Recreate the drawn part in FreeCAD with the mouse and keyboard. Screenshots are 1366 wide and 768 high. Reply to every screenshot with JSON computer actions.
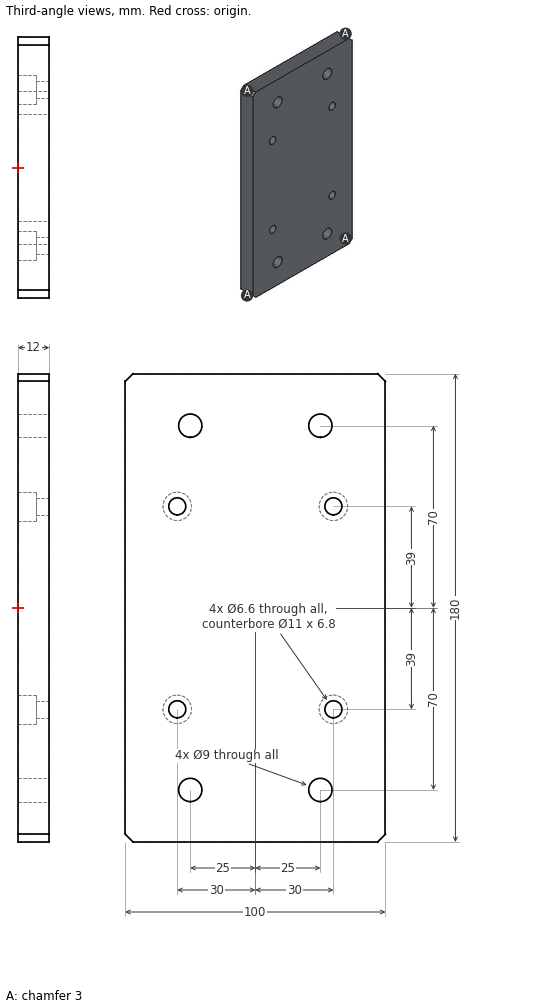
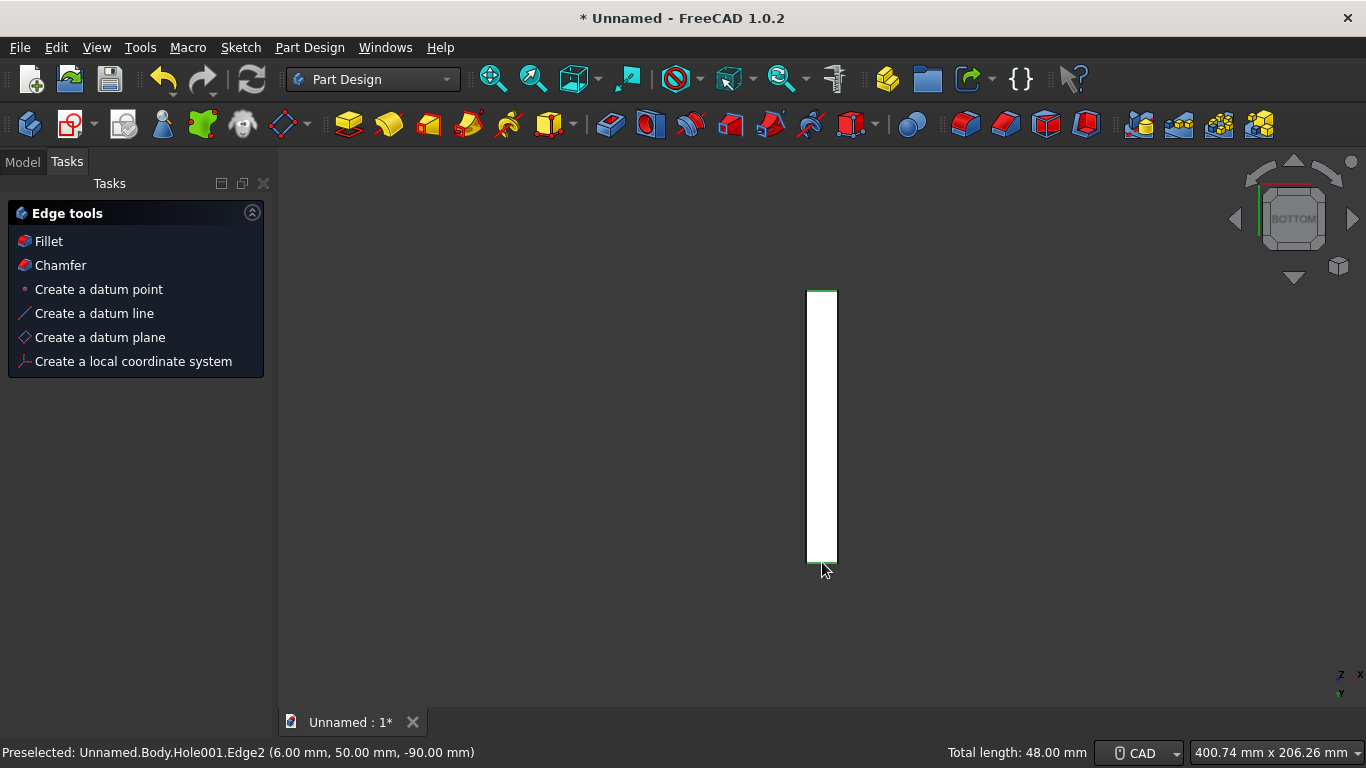
{"action": "left_click", "coordinate": [1006, 124]}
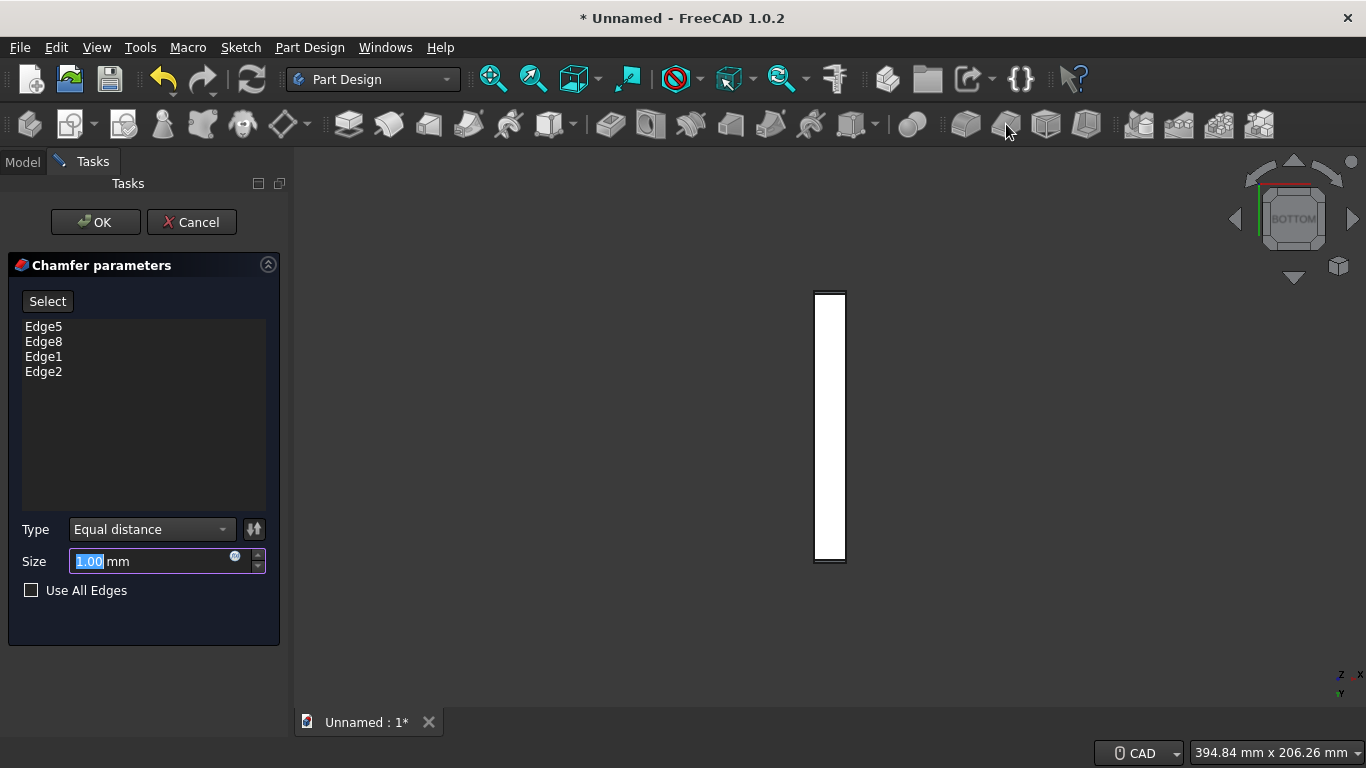
{"action": "type", "text": "3"}
{"action": "key", "text": "Tab"}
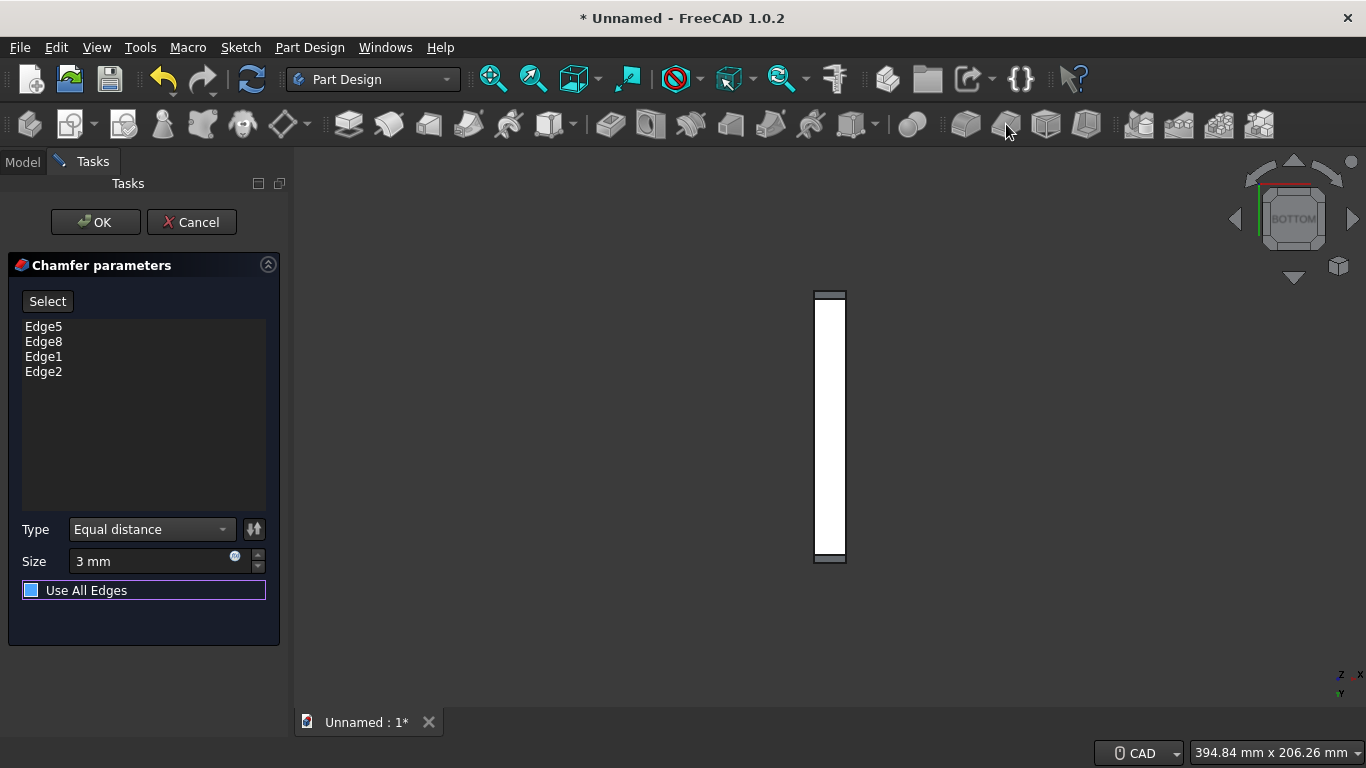
{"action": "left_click", "coordinate": [96, 222]}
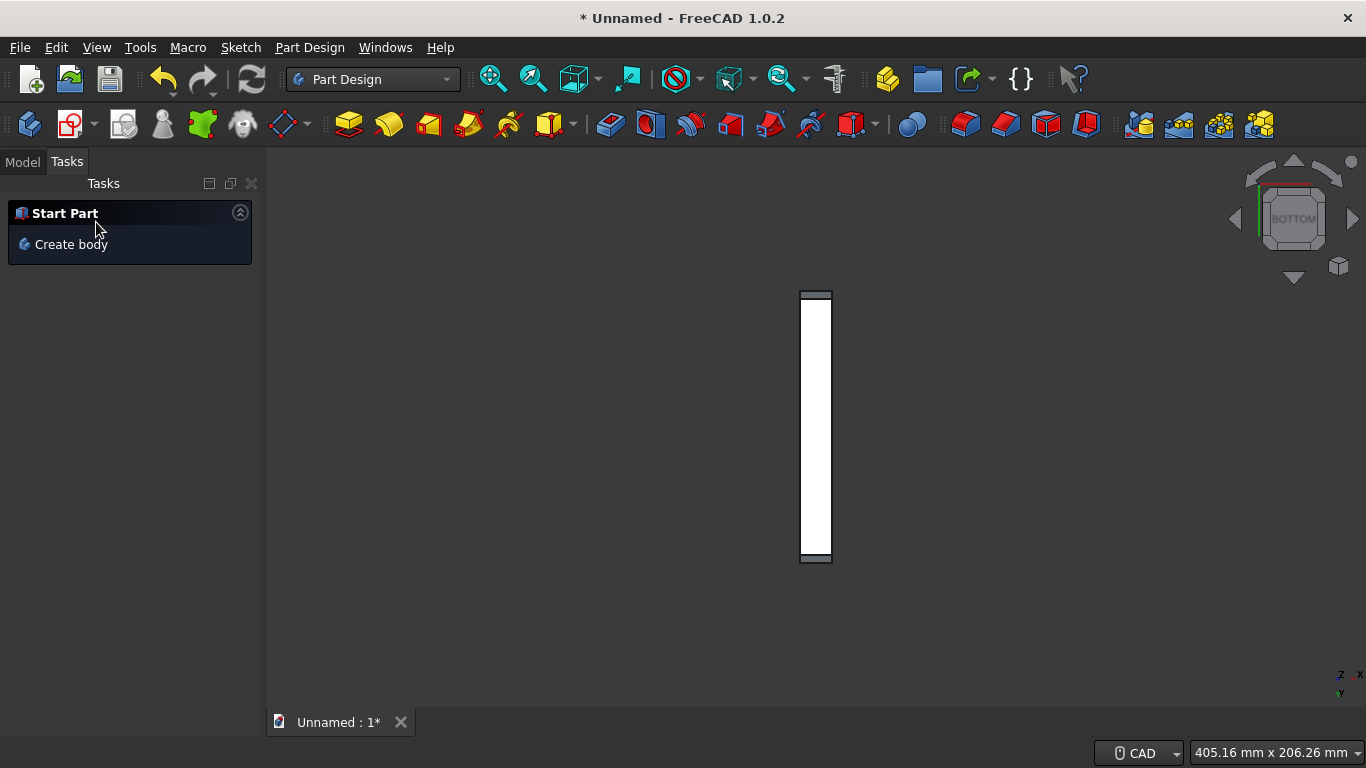
{"action": "key", "text": "0"}